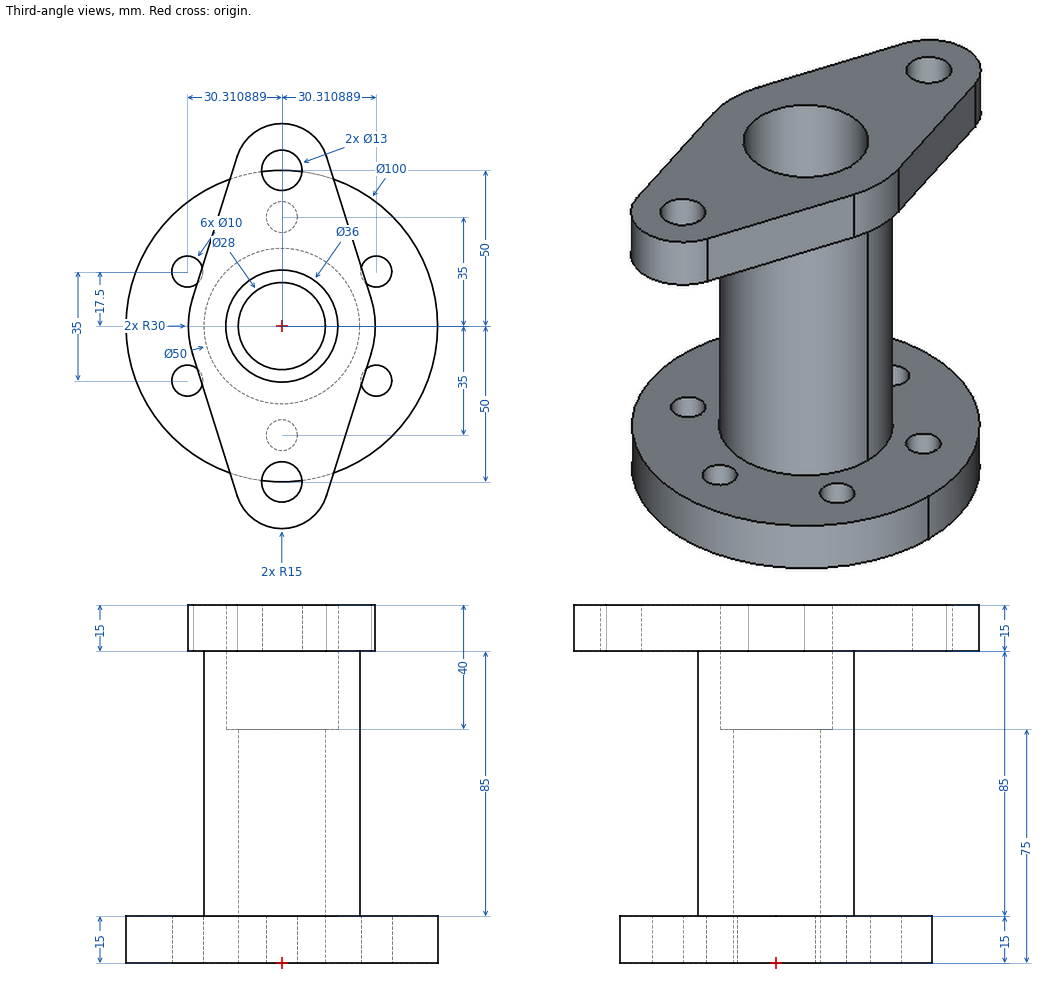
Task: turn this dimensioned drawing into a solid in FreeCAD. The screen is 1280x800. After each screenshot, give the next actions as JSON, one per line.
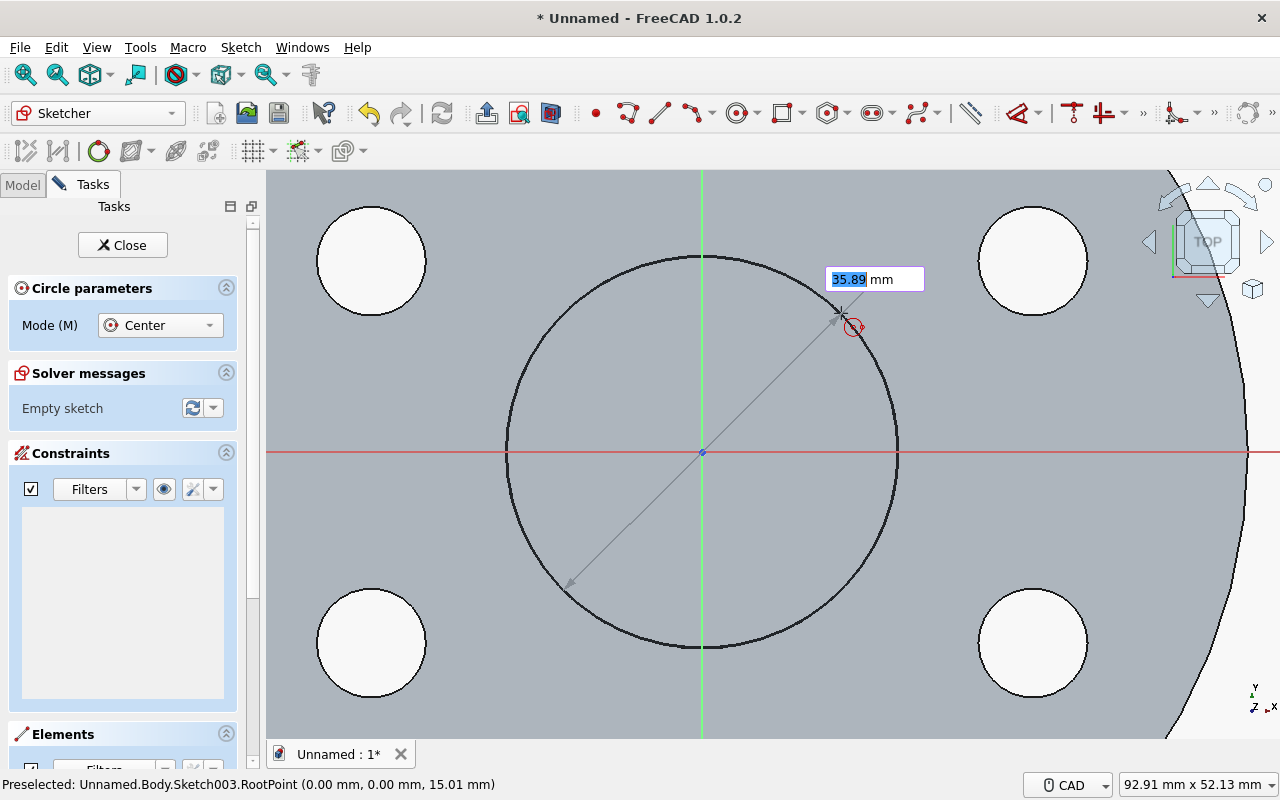
{"action": "type", "text": "36"}
{"action": "key", "text": "Return"}
{"action": "key", "text": "Escape"}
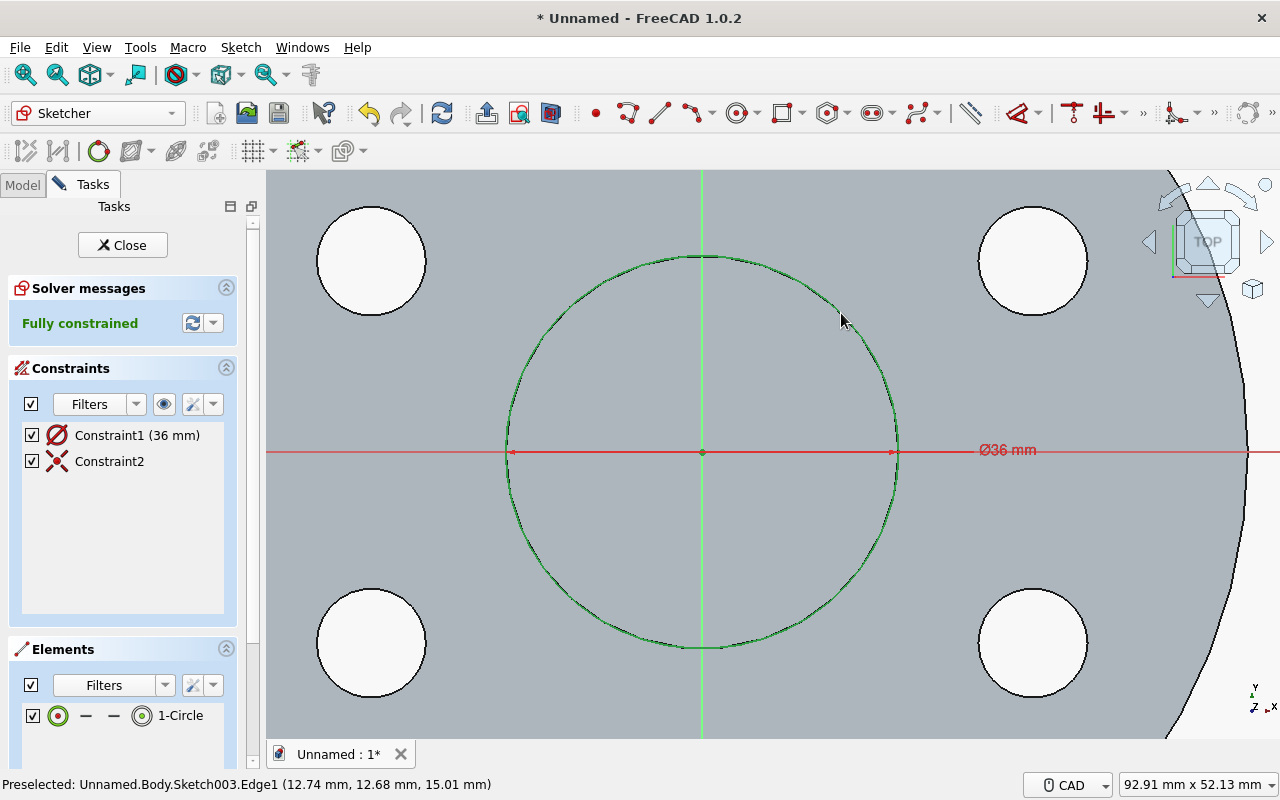
{"action": "left_click", "coordinate": [123, 245]}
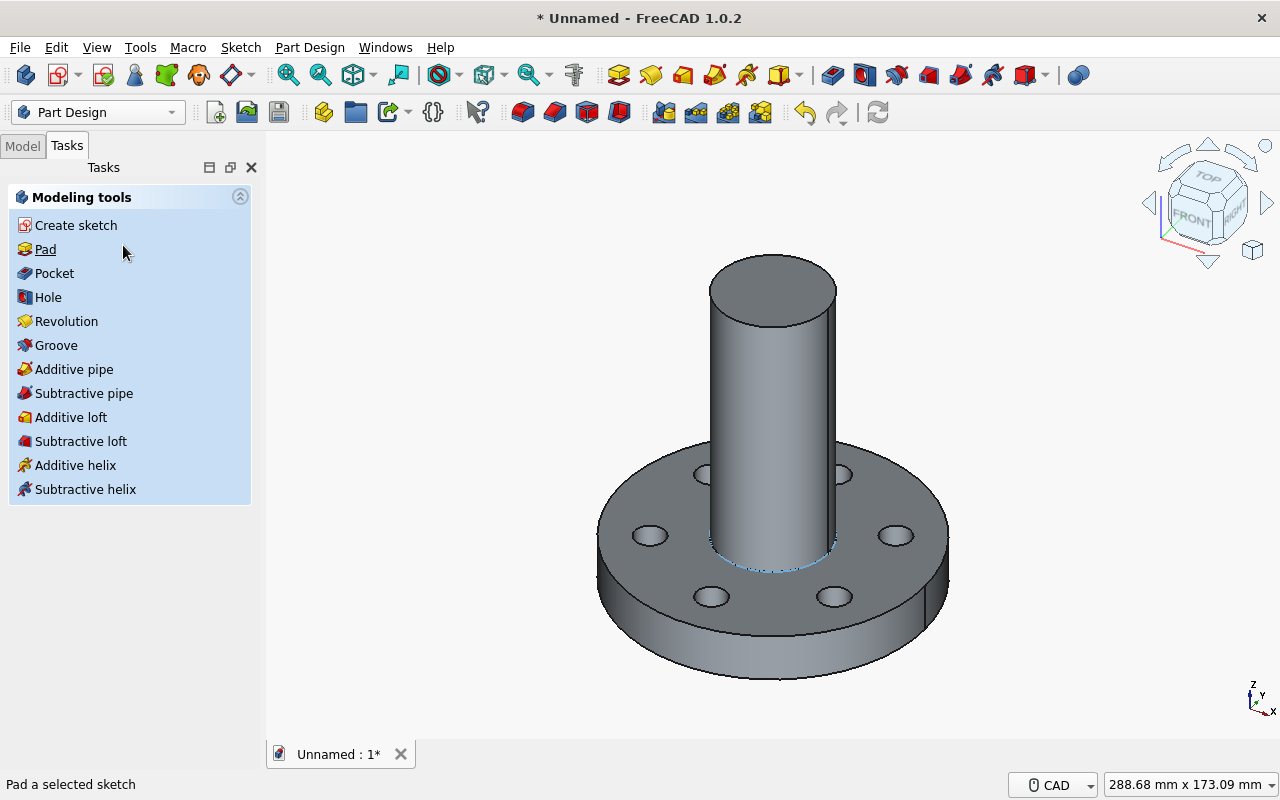
{"action": "left_click", "coordinate": [834, 76]}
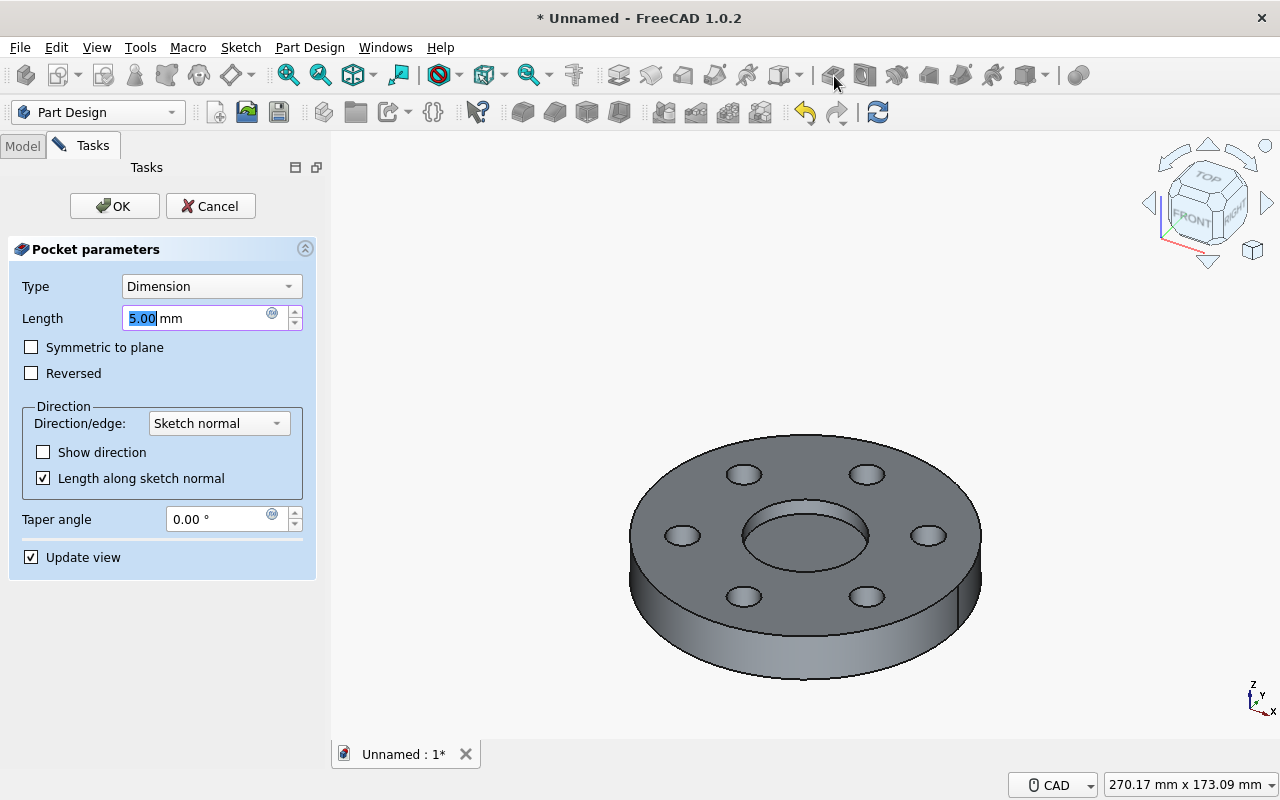
{"action": "type", "text": "85"}
{"action": "key", "text": "Tab"}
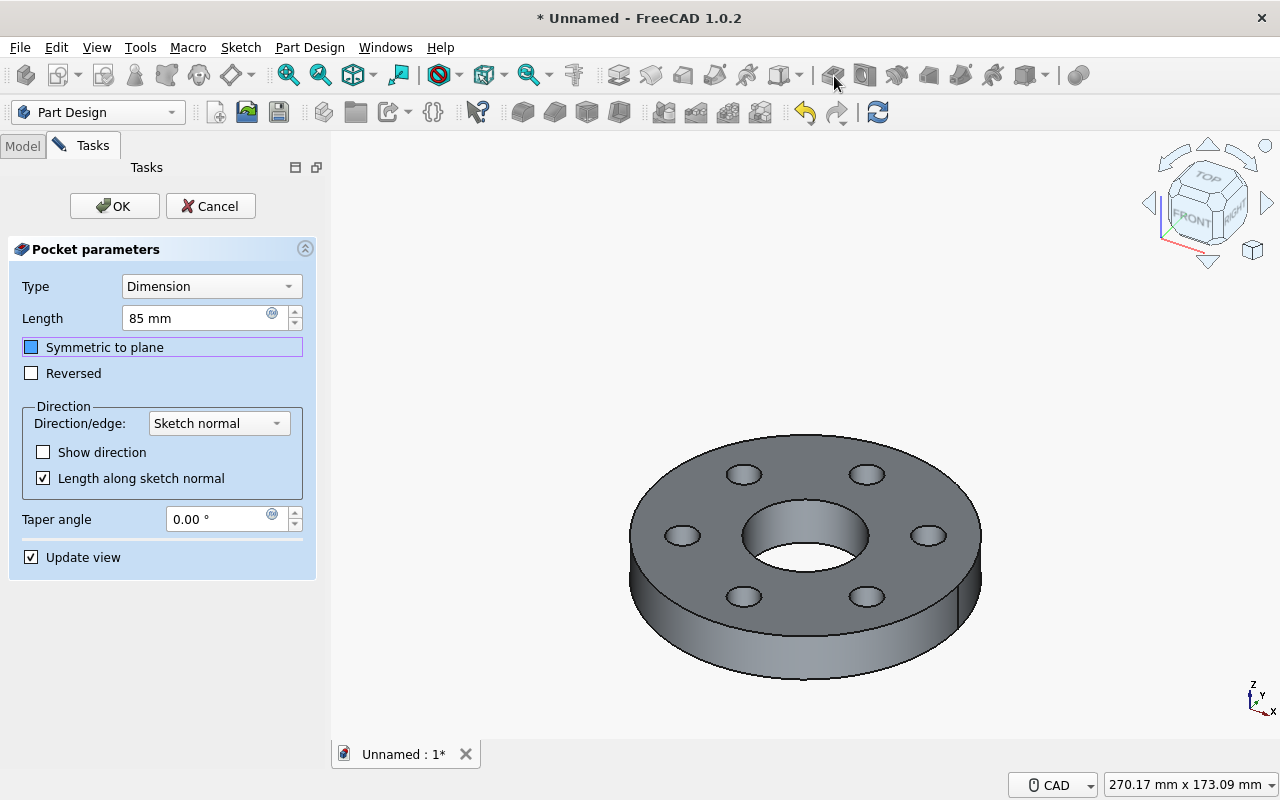
{"action": "left_click", "coordinate": [30, 373]}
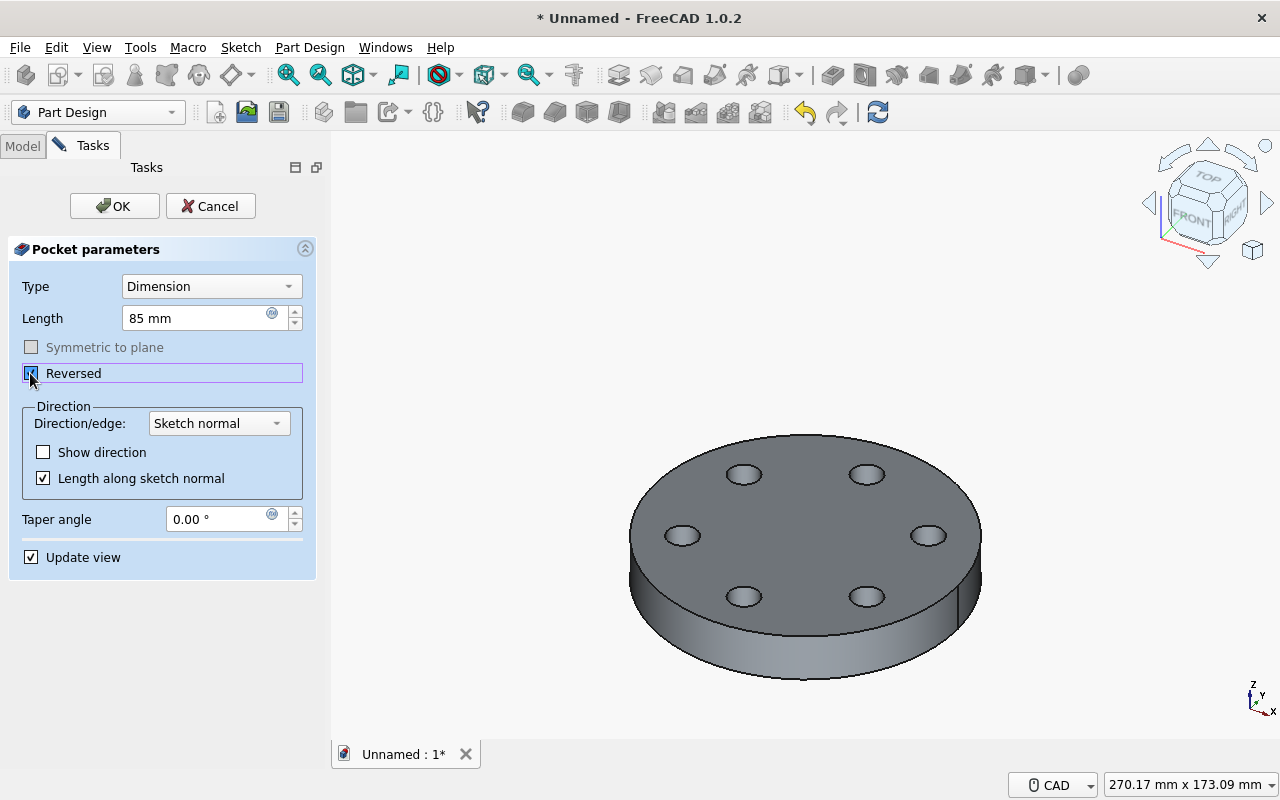
{"action": "left_click", "coordinate": [115, 206]}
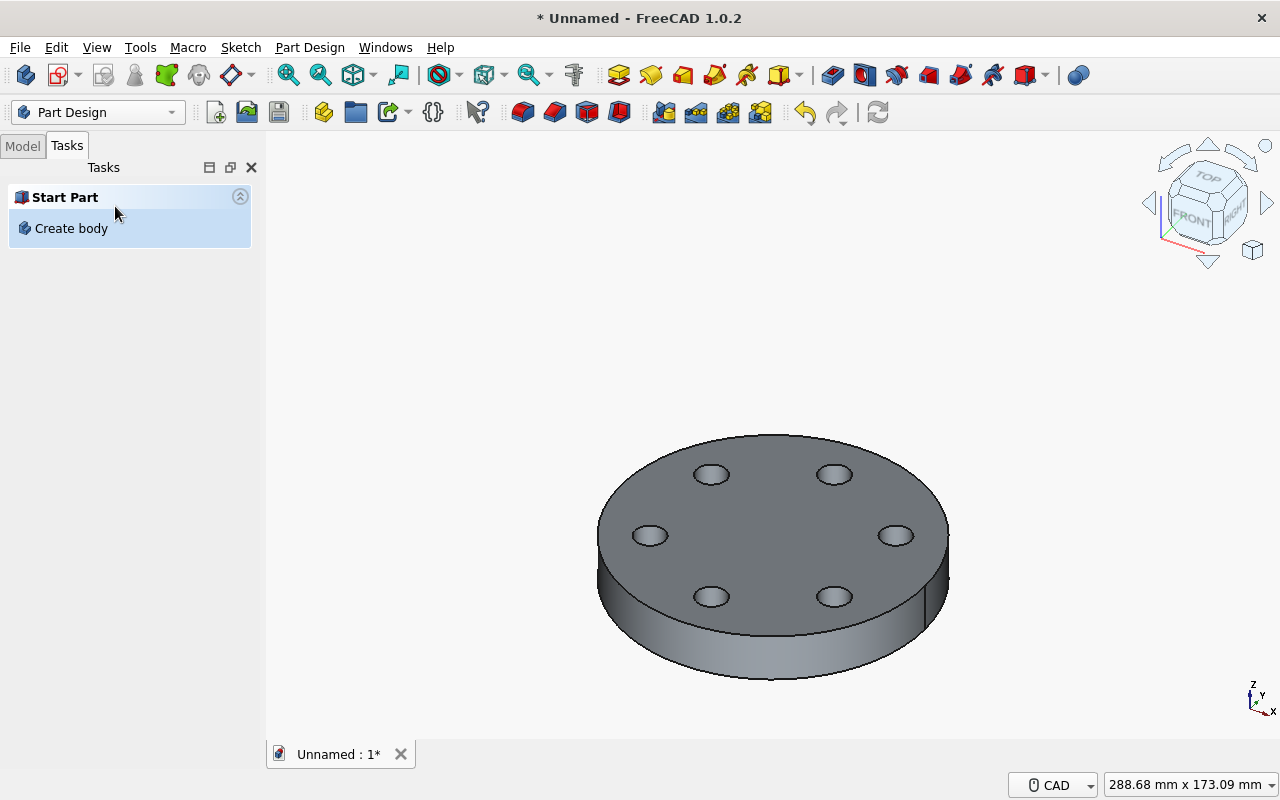
{"action": "left_click", "coordinate": [773, 535]}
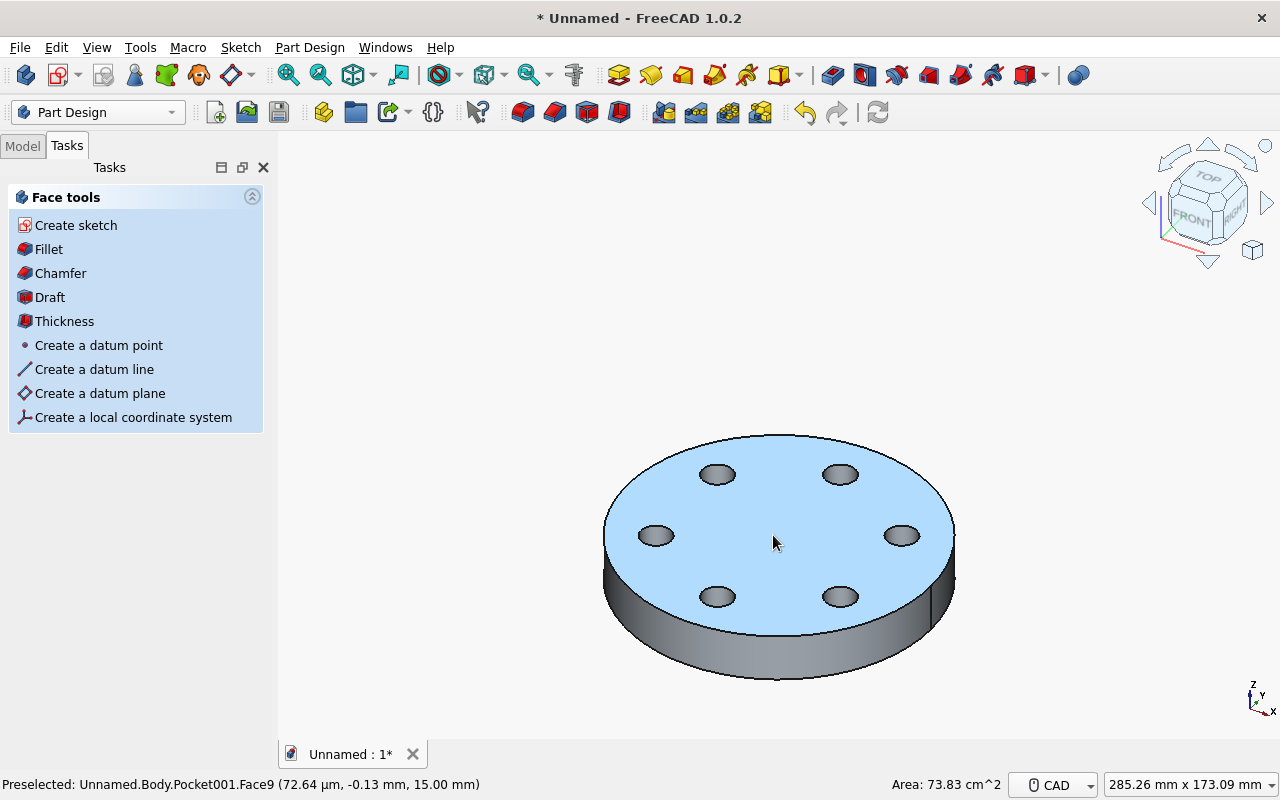
{"action": "left_click", "coordinate": [58, 76]}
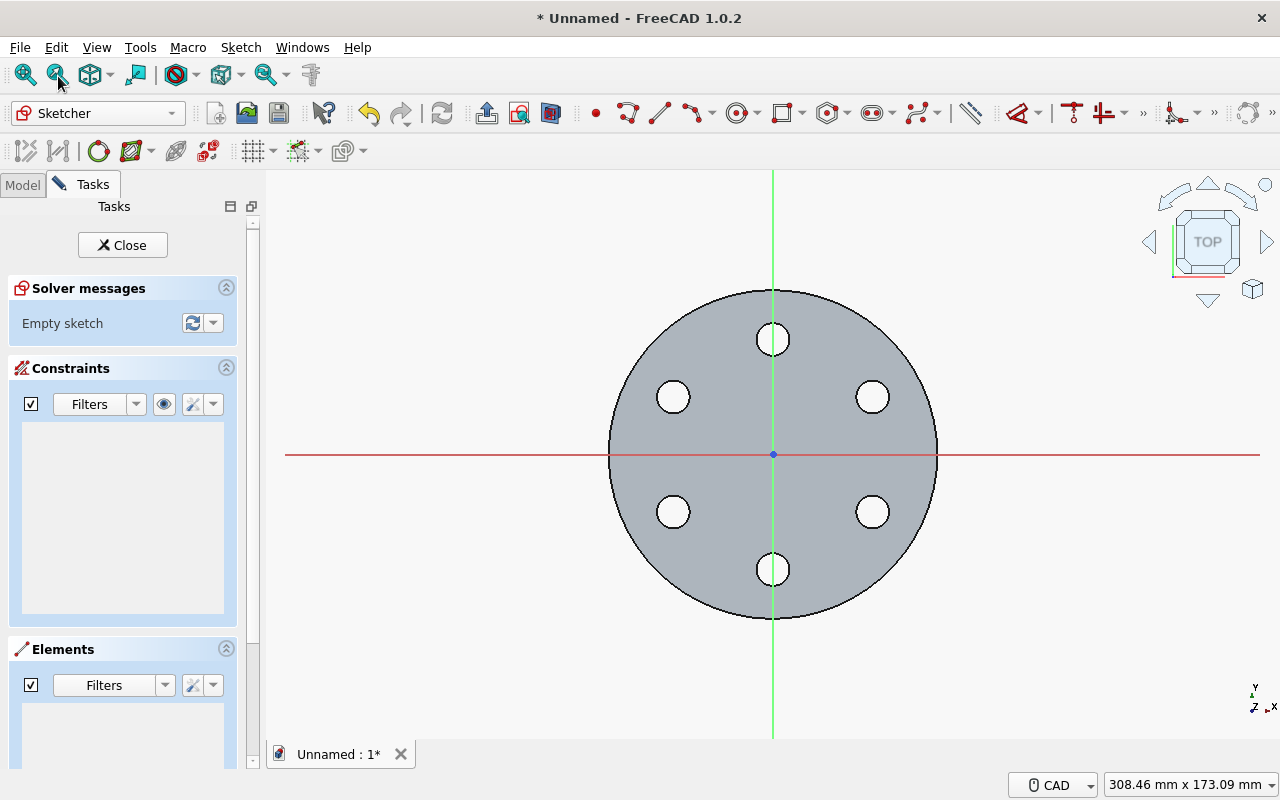
{"action": "scroll", "coordinate": [829, 455], "scroll_direction": "up", "scroll_amount": 4}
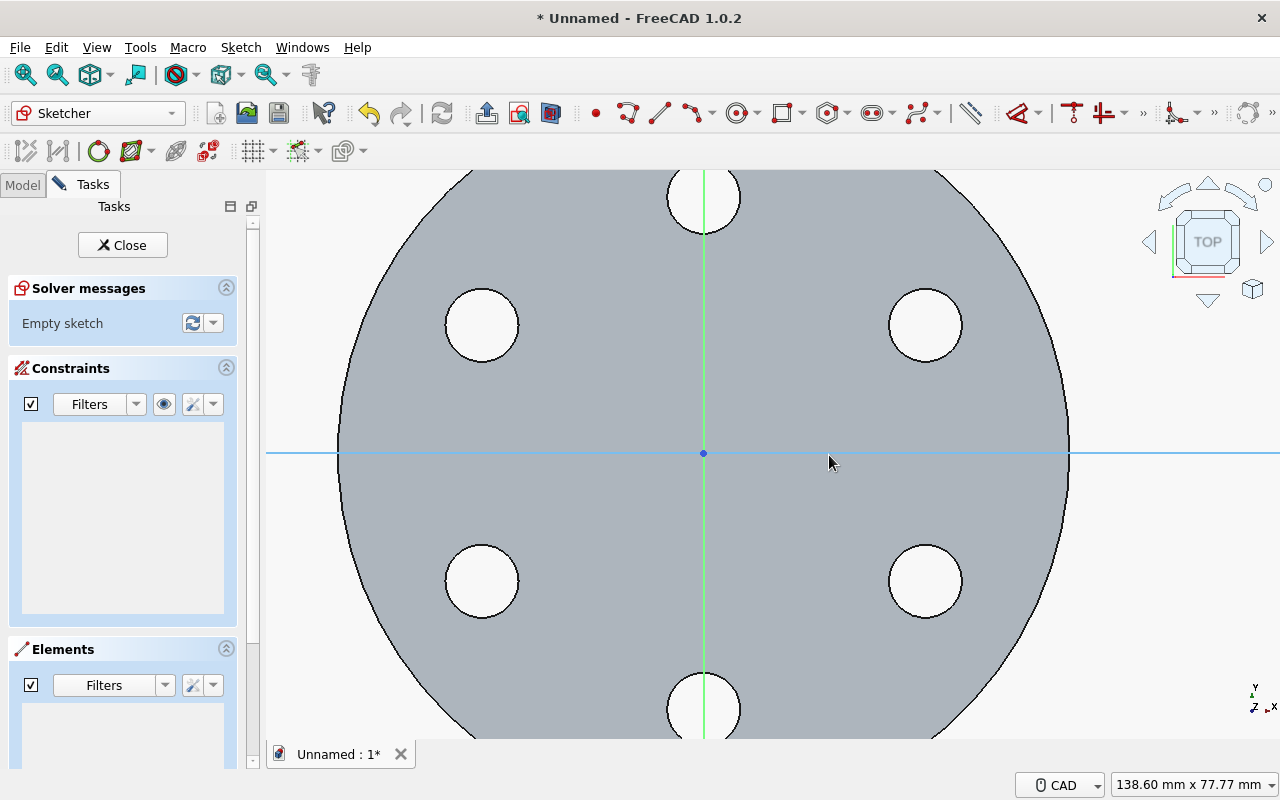
{"action": "left_click", "coordinate": [738, 114]}